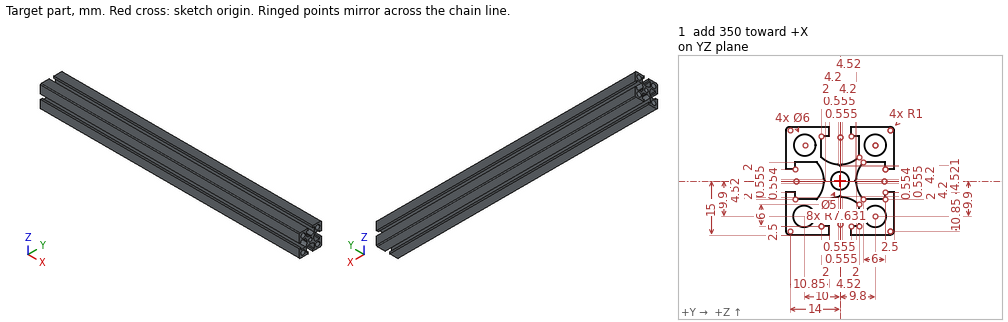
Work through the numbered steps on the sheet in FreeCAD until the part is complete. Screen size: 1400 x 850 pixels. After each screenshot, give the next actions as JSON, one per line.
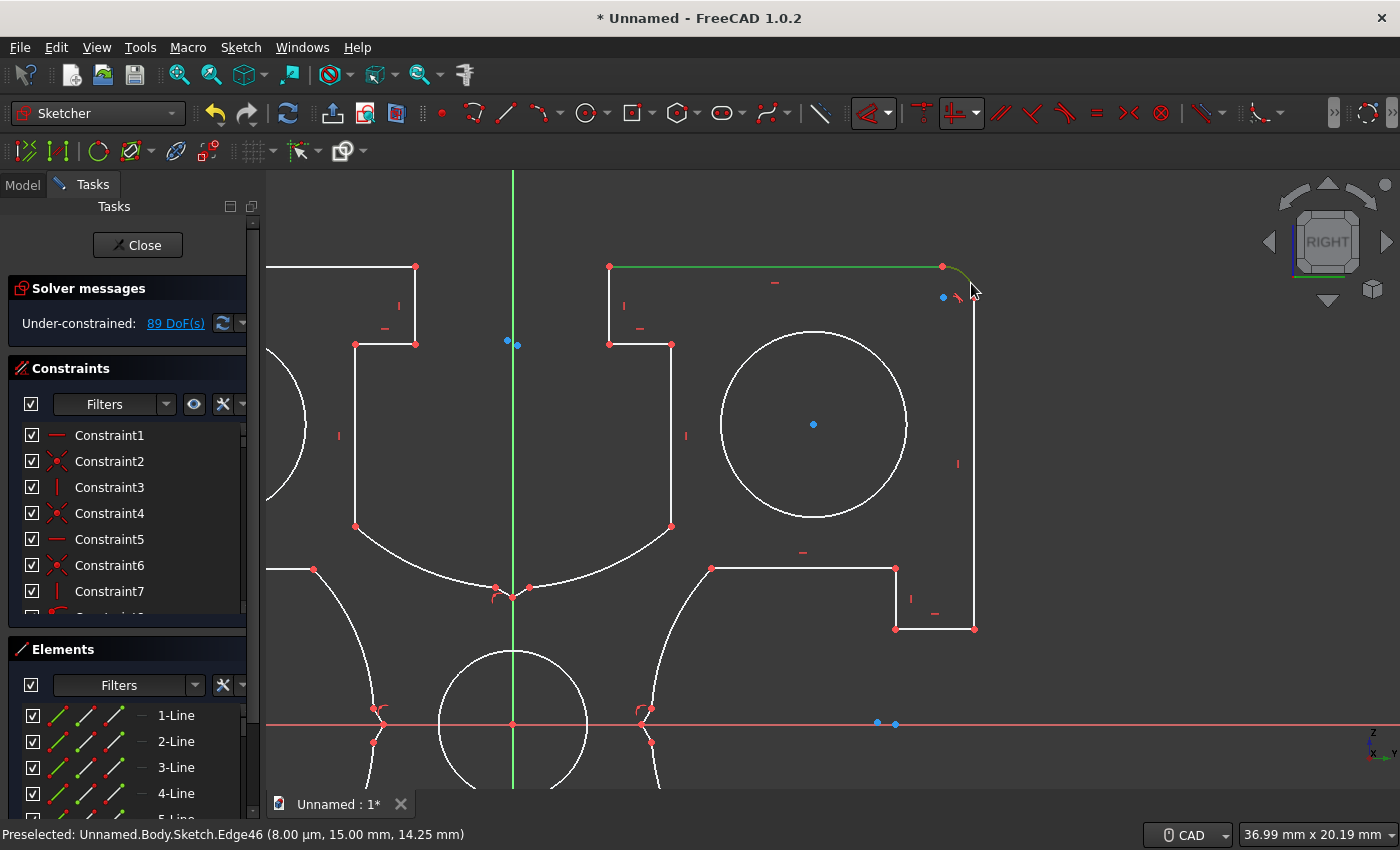
{"action": "left_click", "coordinate": [1066, 114]}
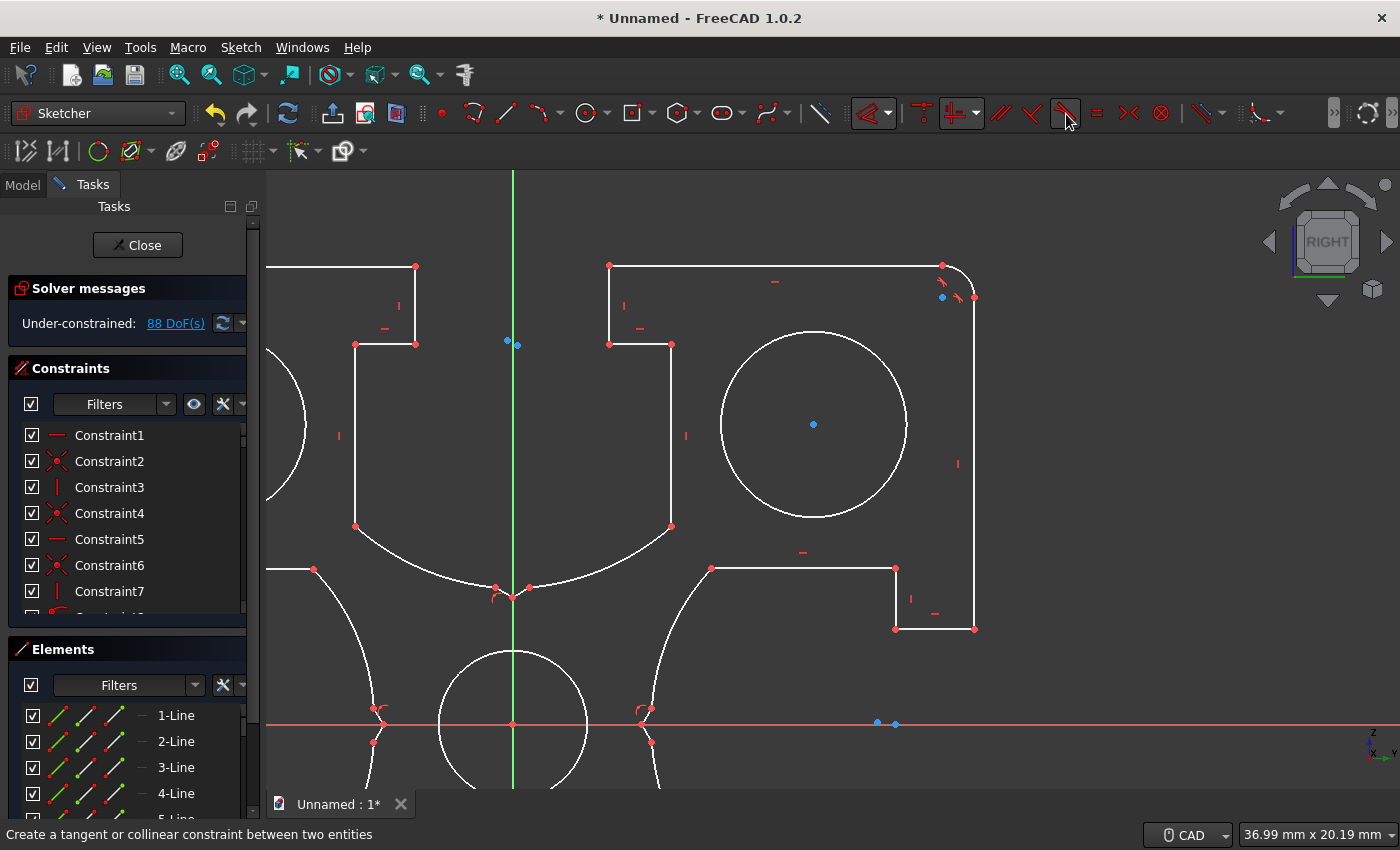
{"action": "left_click", "coordinate": [316, 267]}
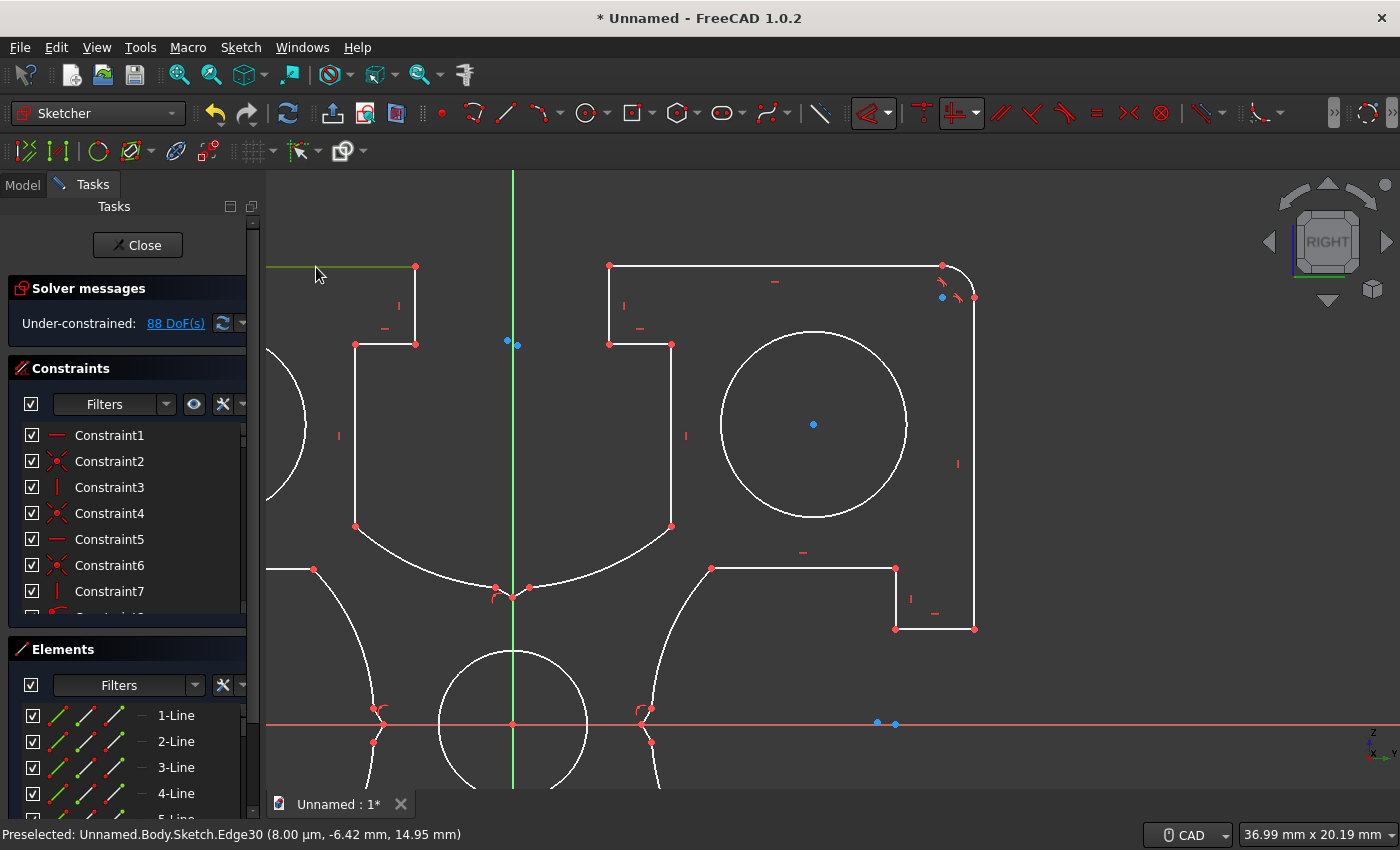
{"action": "scroll", "coordinate": [970, 279], "scroll_direction": "down", "scroll_amount": 4}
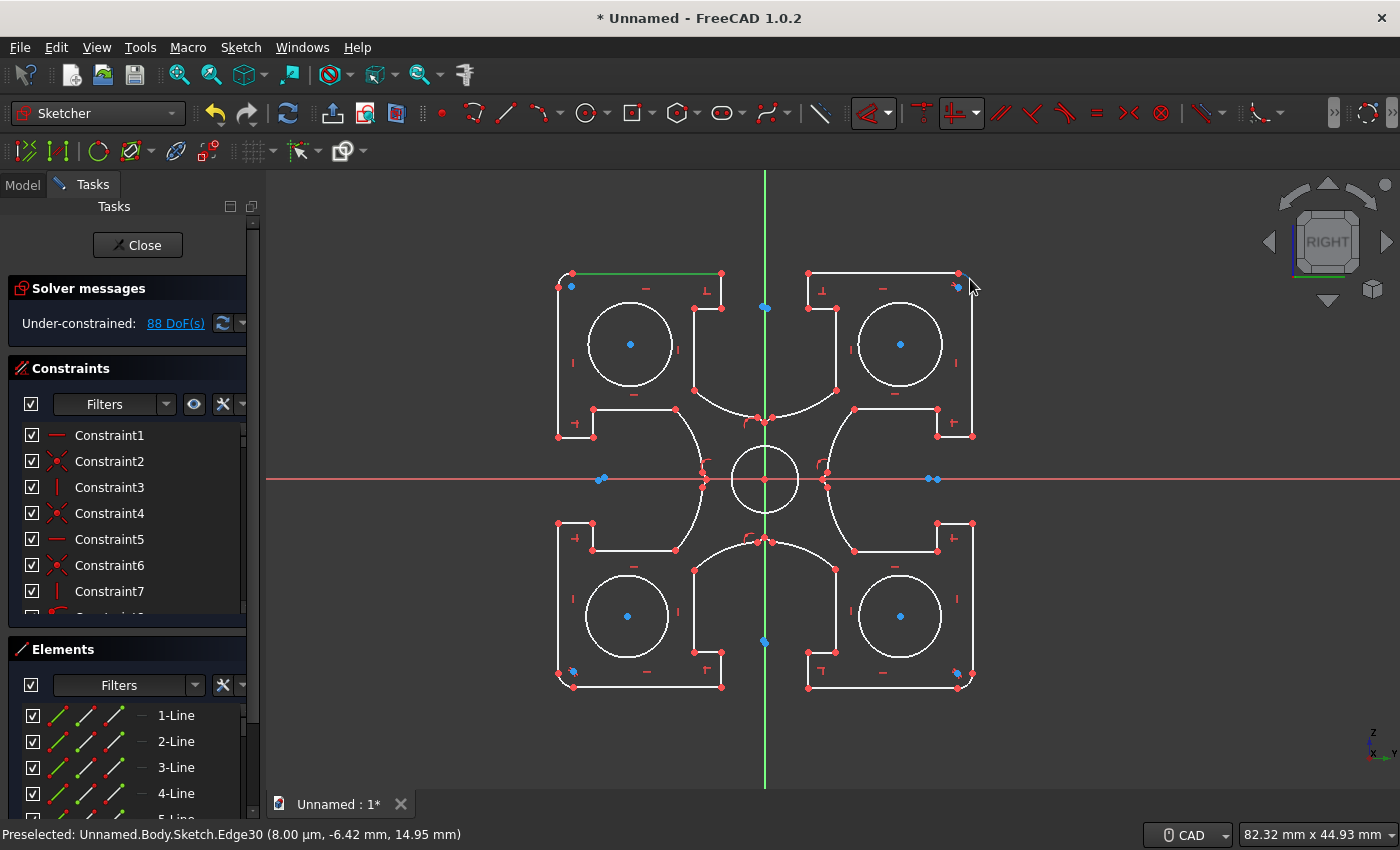
{"action": "scroll", "coordinate": [566, 275], "scroll_direction": "up", "scroll_amount": 4}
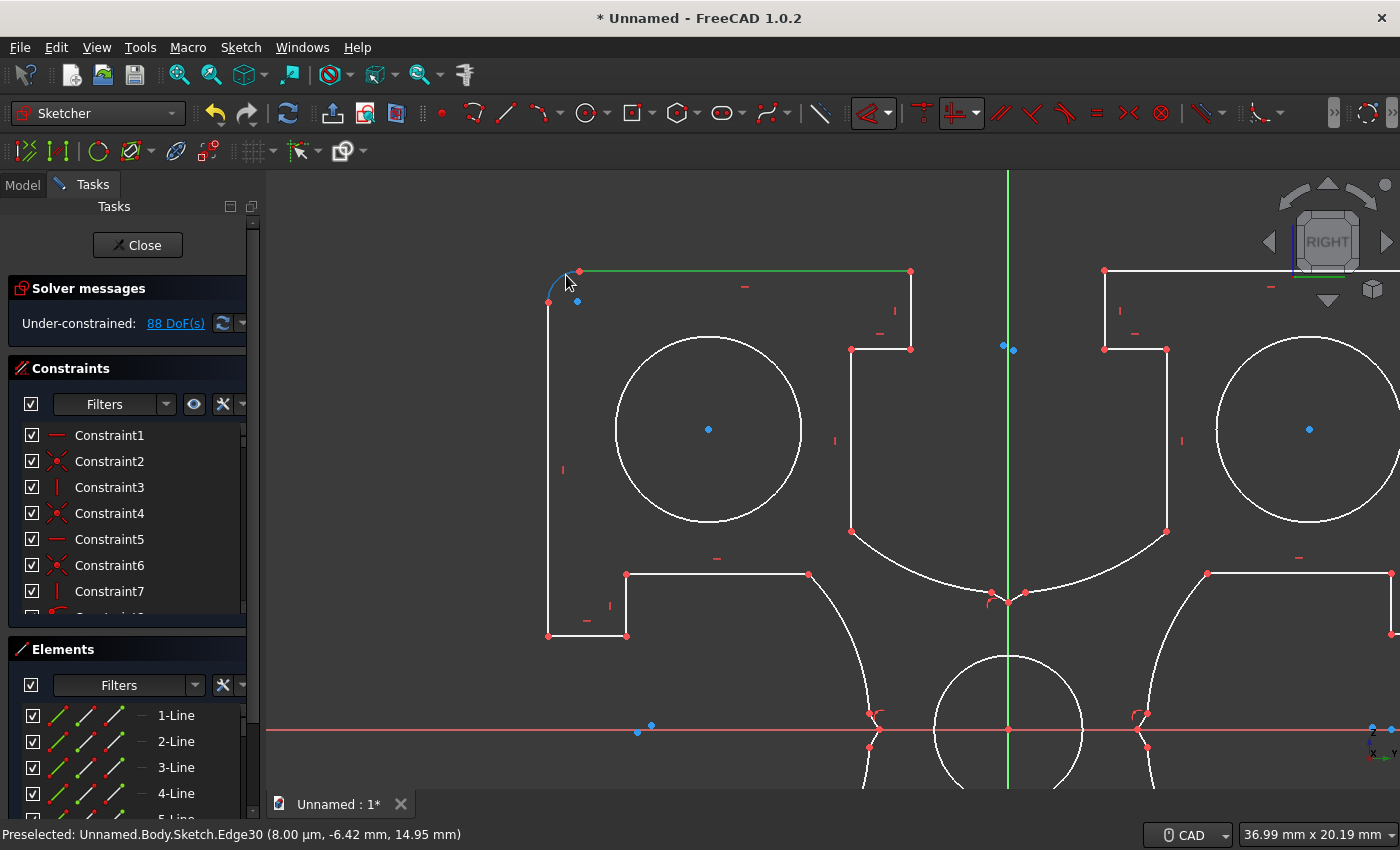
{"action": "left_click", "coordinate": [565, 274]}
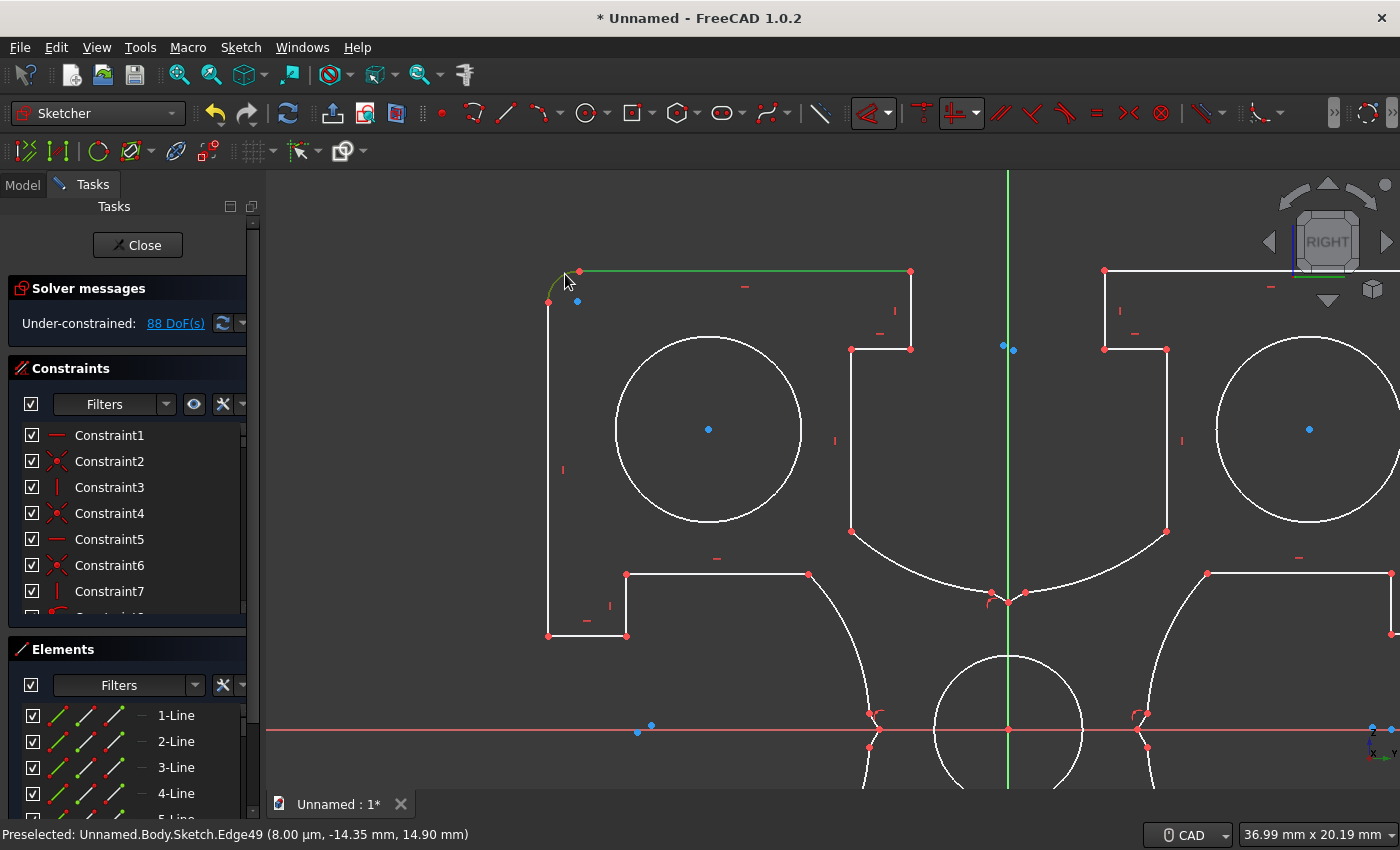
{"action": "key", "text": "t"}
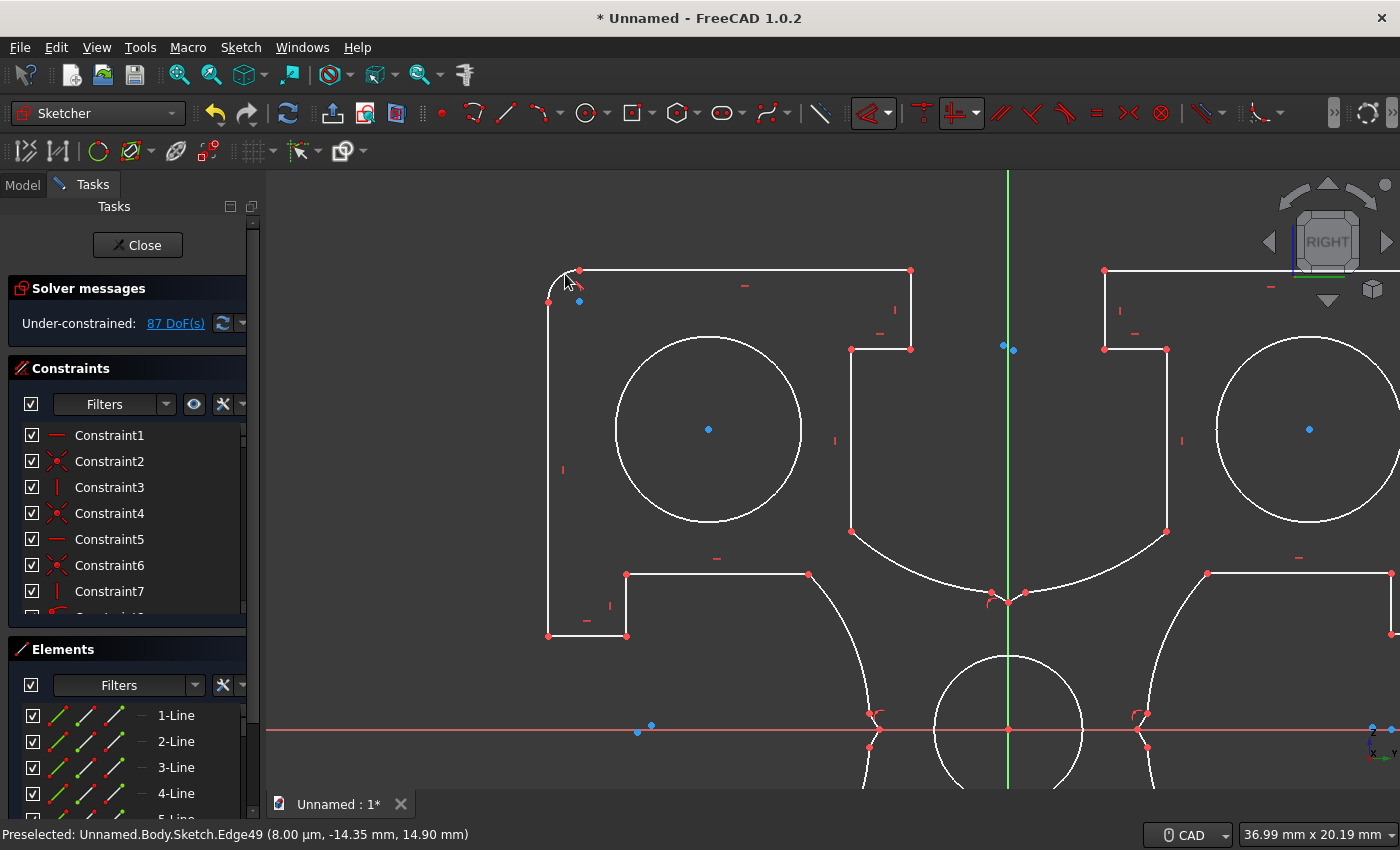
{"action": "left_click", "coordinate": [548, 403]}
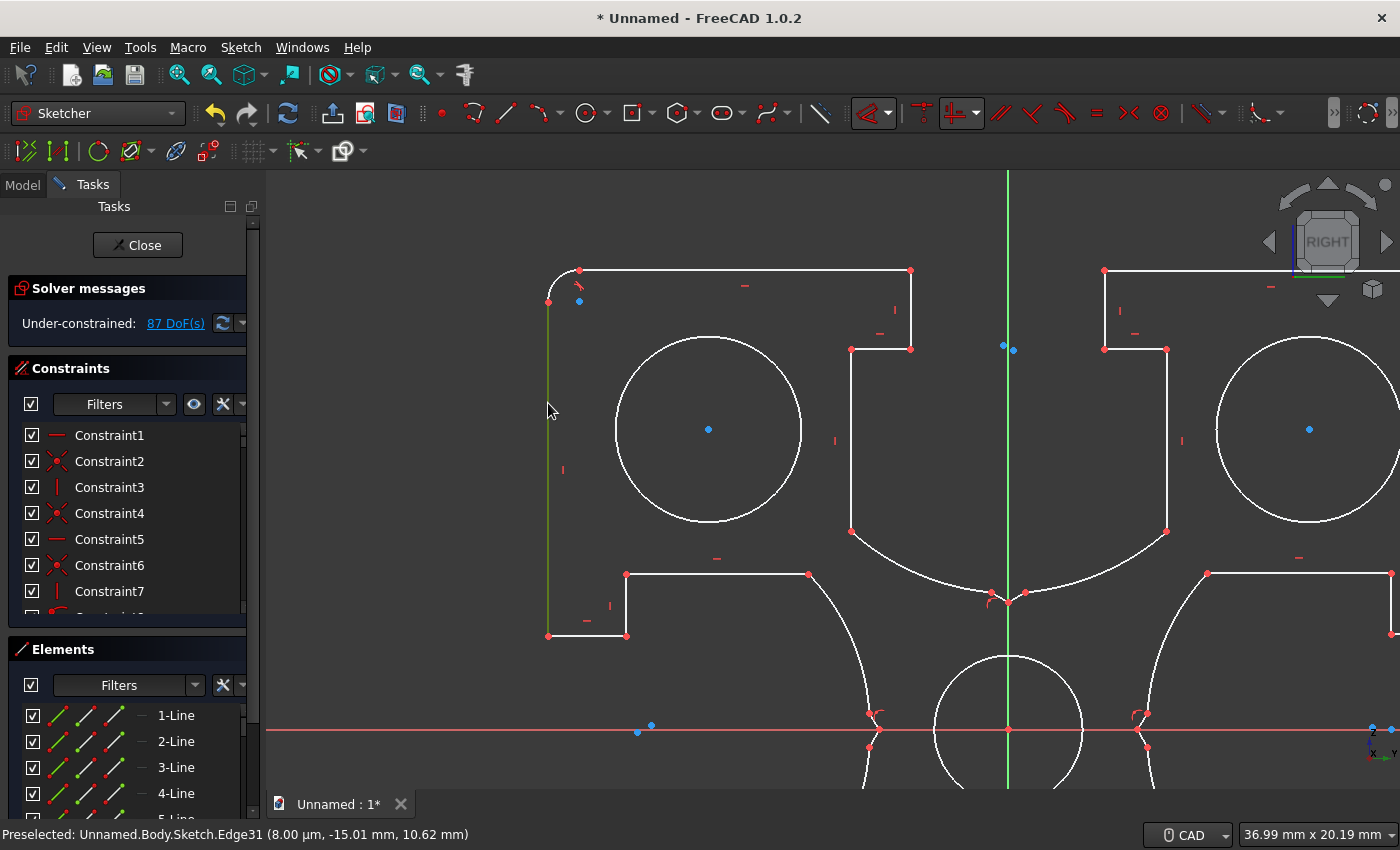
{"action": "left_click", "coordinate": [565, 274]}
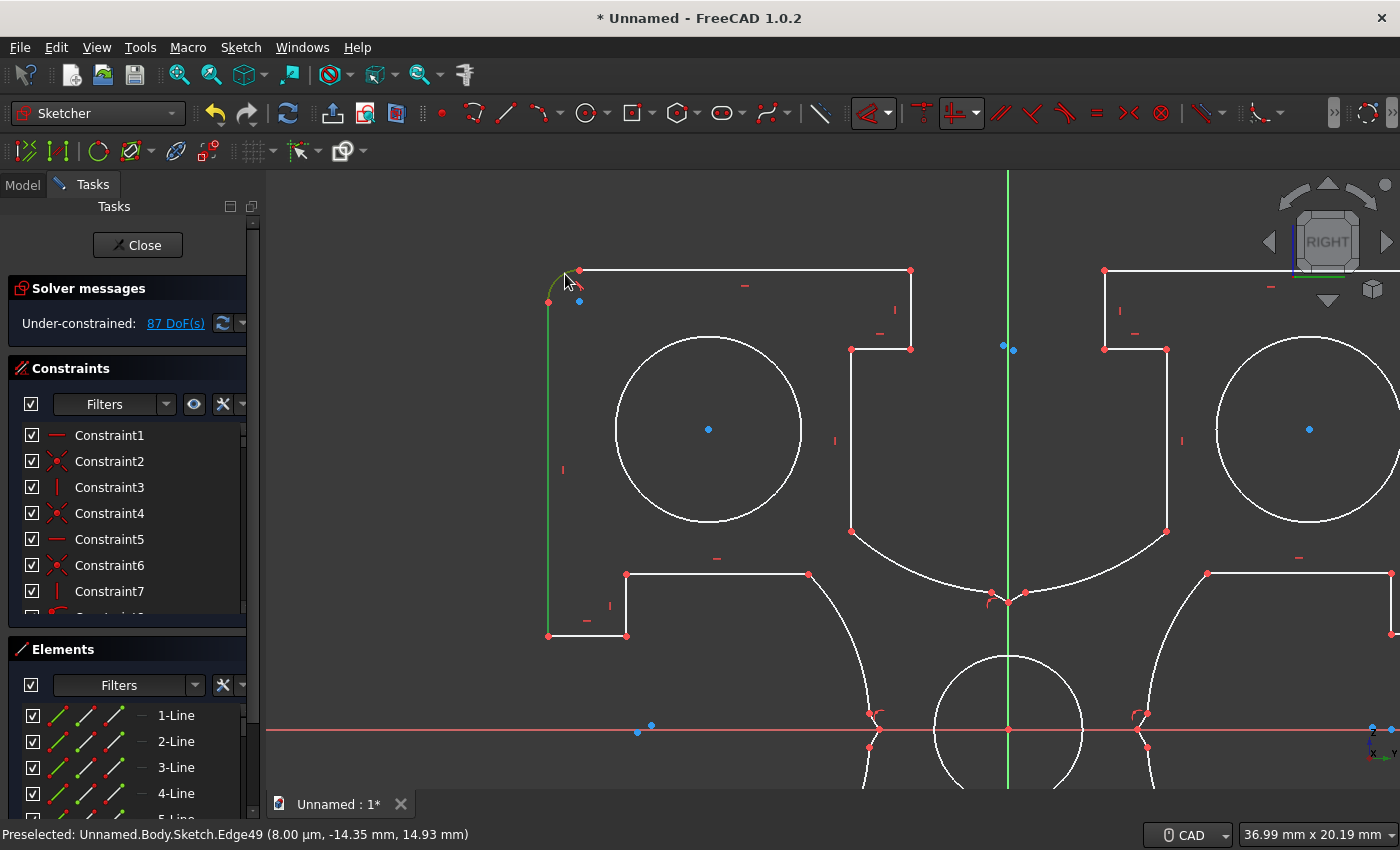
{"action": "left_click", "coordinate": [1066, 114]}